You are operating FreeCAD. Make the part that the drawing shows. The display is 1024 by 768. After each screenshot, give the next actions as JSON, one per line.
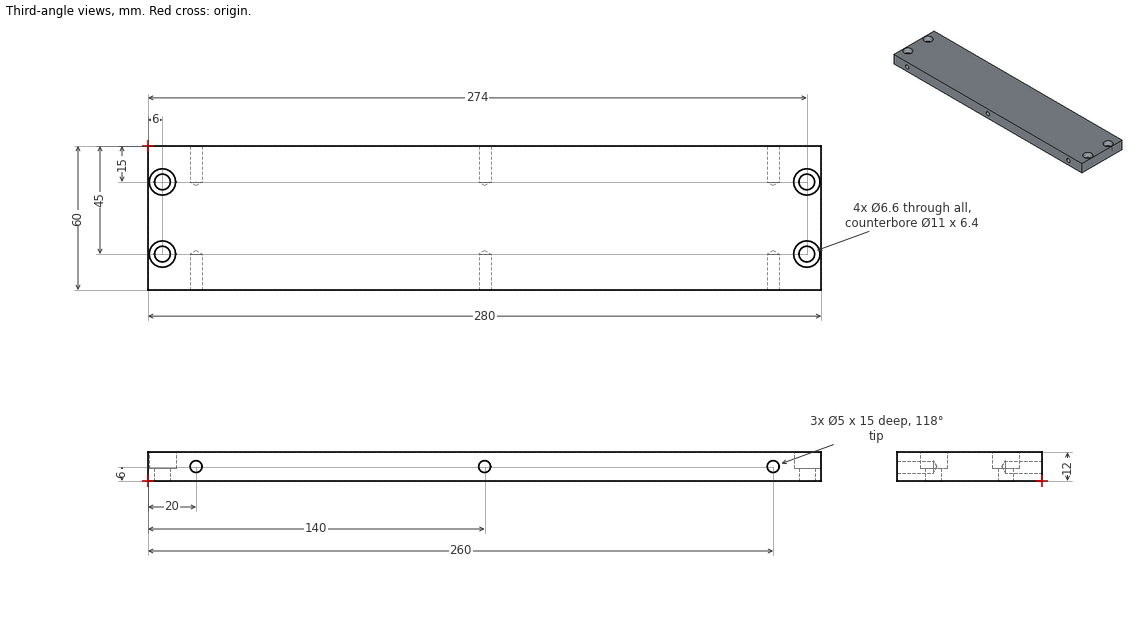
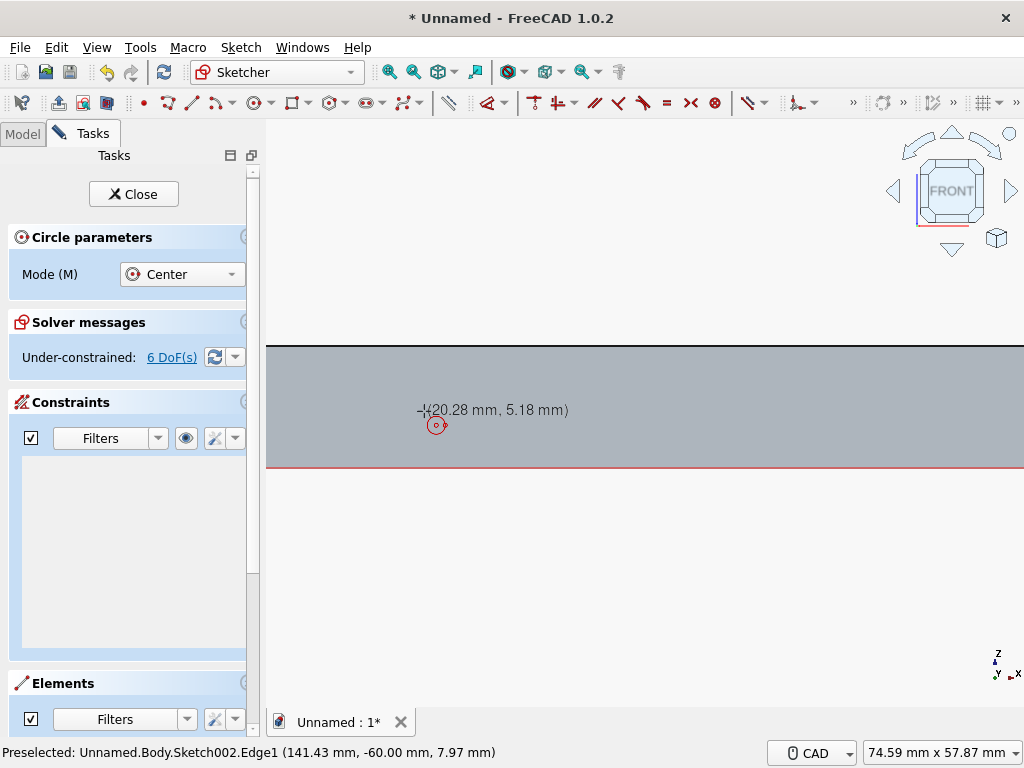
{"action": "scroll", "coordinate": [424, 411], "scroll_direction": "down", "scroll_amount": 10}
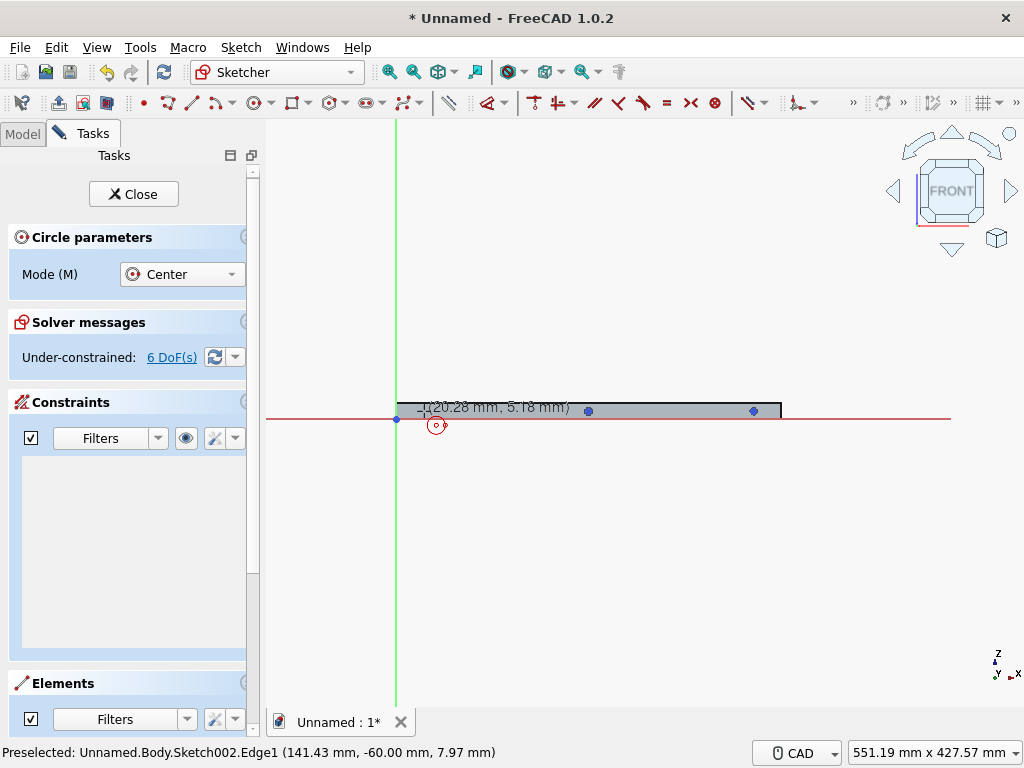
{"action": "scroll", "coordinate": [424, 411], "scroll_direction": "up", "scroll_amount": 4}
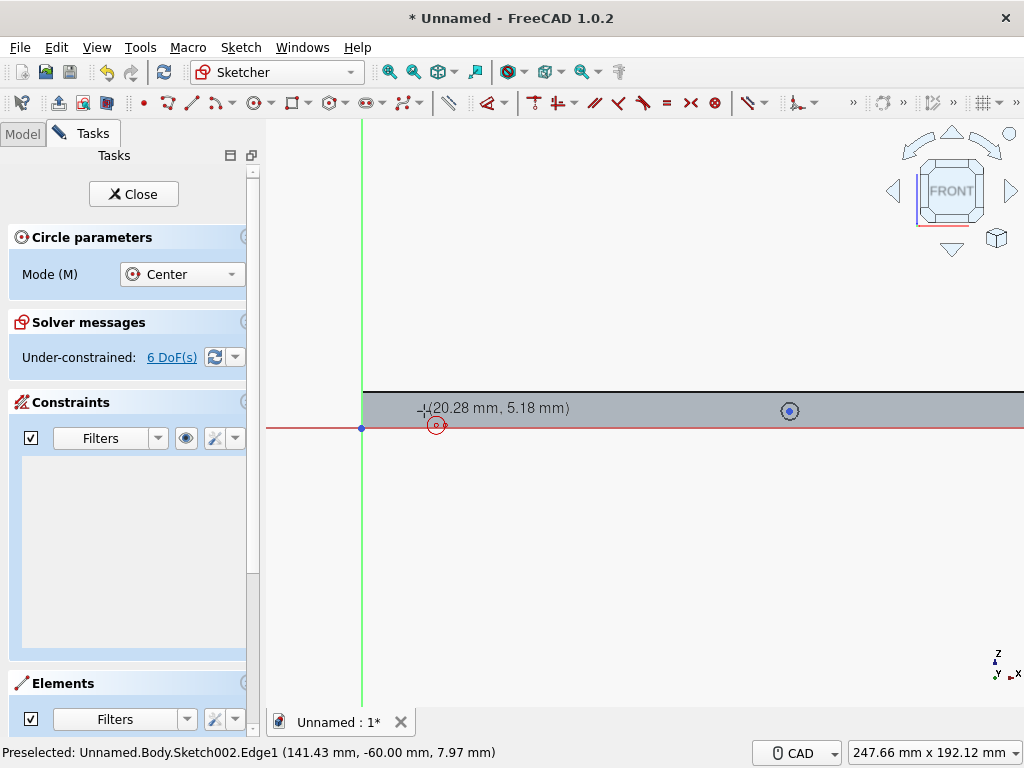
{"action": "left_click", "coordinate": [423, 410]}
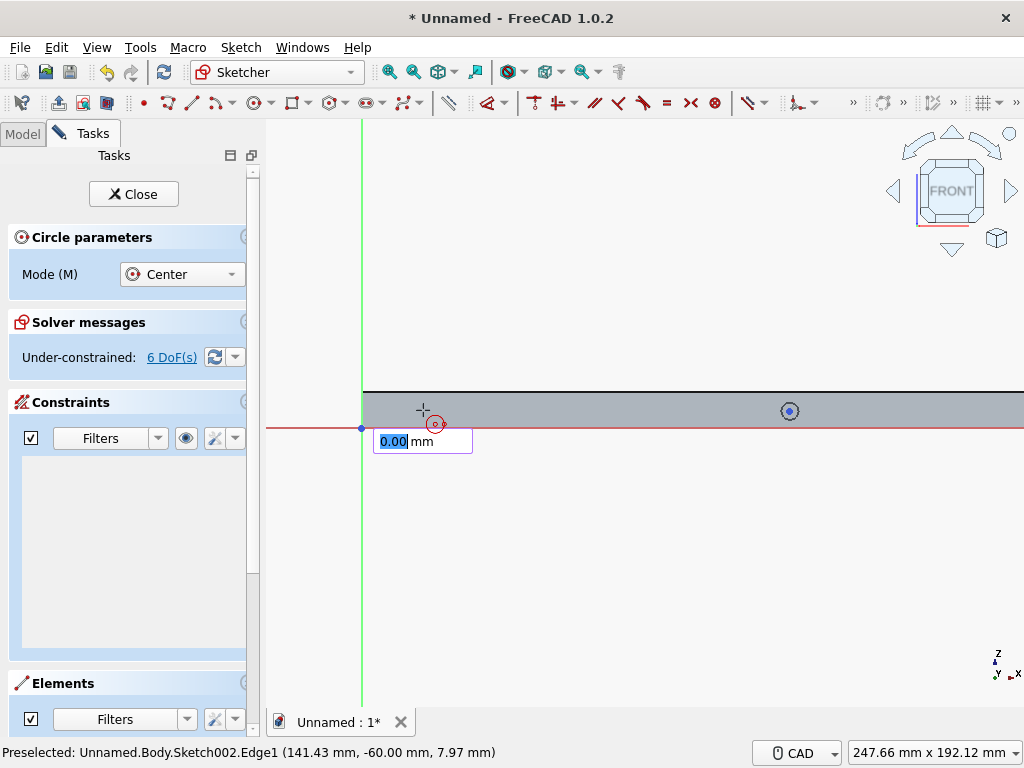
{"action": "scroll", "coordinate": [428, 405], "scroll_direction": "up", "scroll_amount": 4}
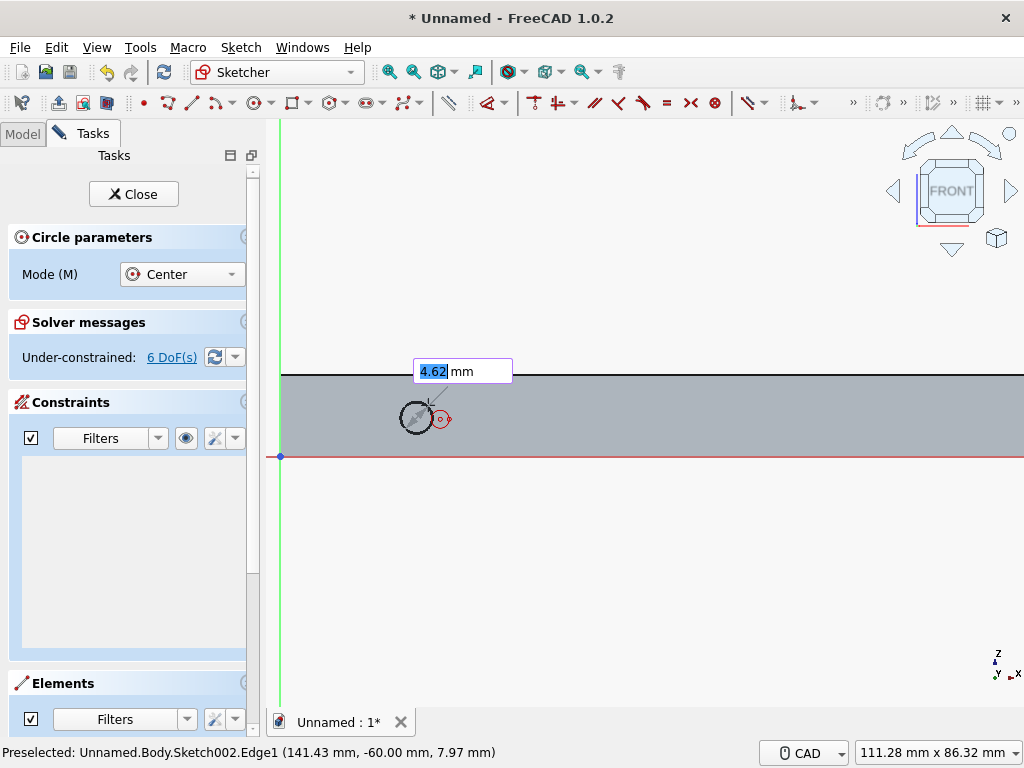
{"action": "left_click", "coordinate": [428, 404]}
{"action": "key", "text": "Escape"}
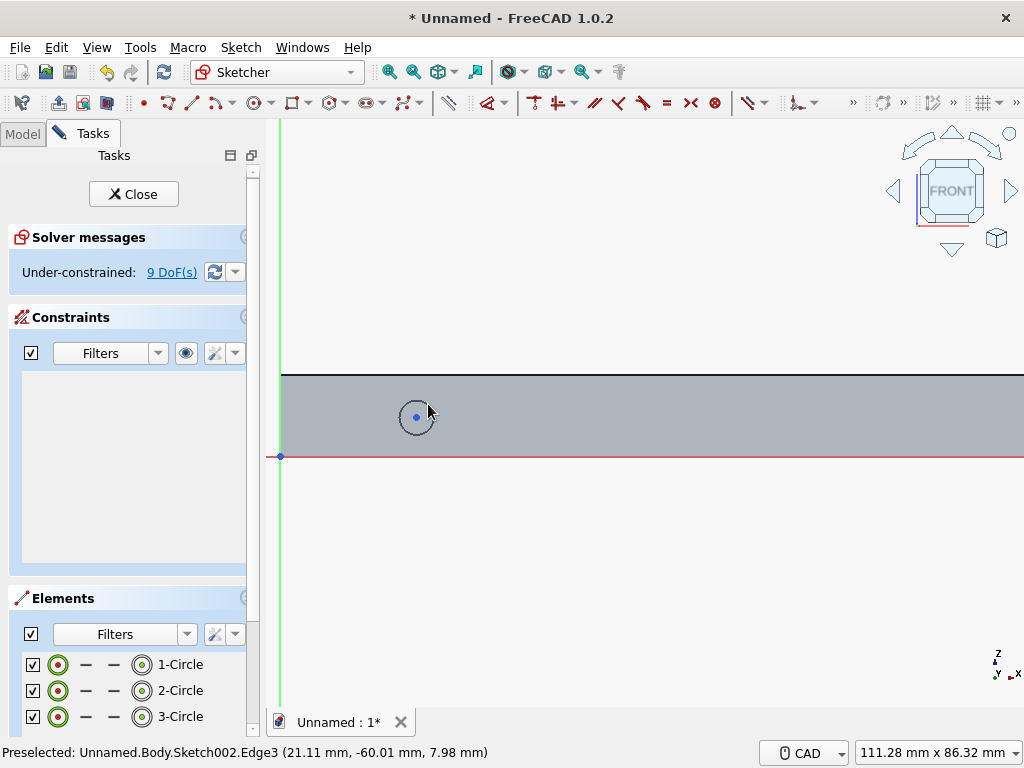
{"action": "scroll", "coordinate": [425, 409], "scroll_direction": "down", "scroll_amount": 8}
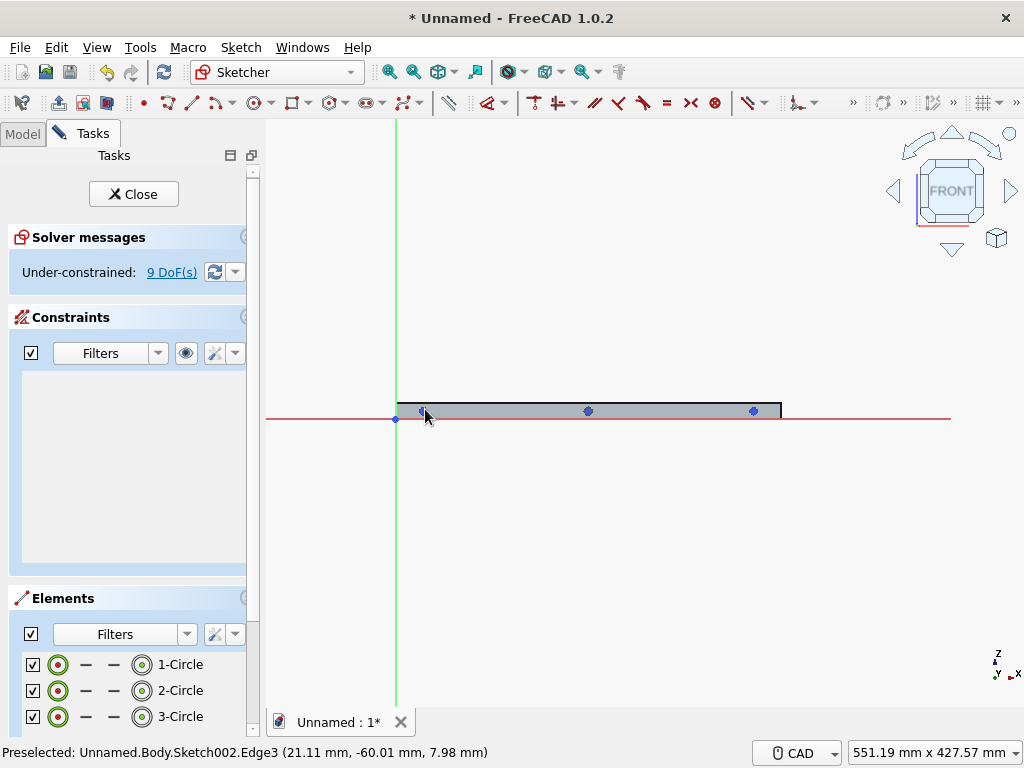
{"action": "scroll", "coordinate": [756, 409], "scroll_direction": "up", "scroll_amount": 8}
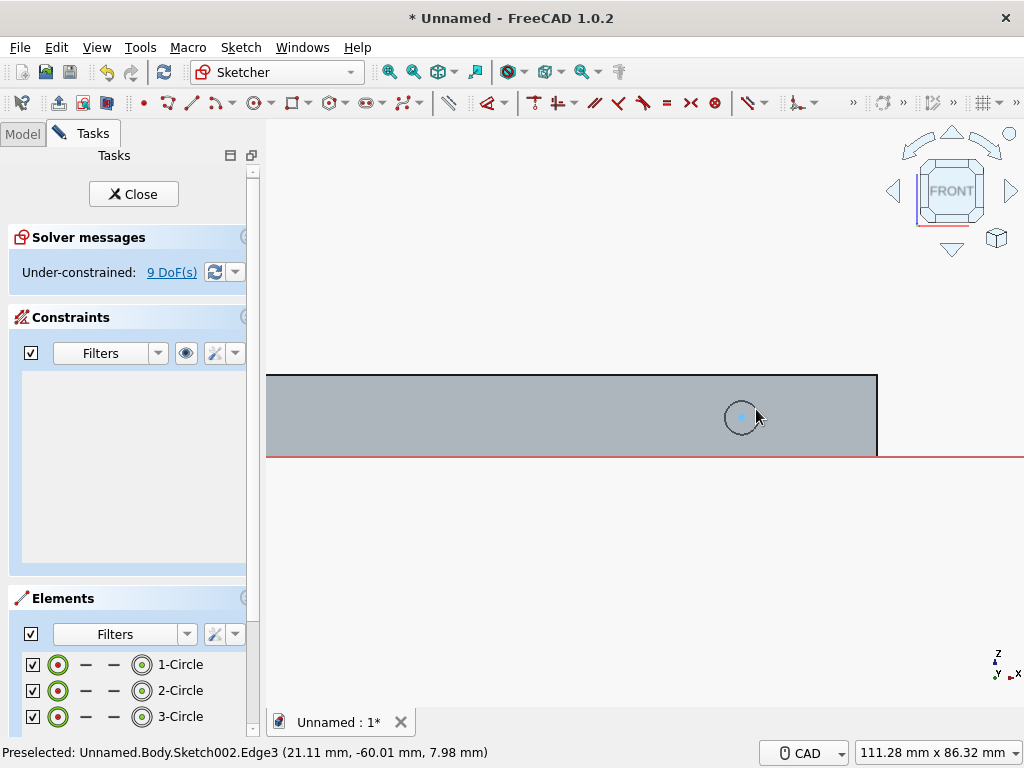
{"action": "left_click", "coordinate": [754, 406]}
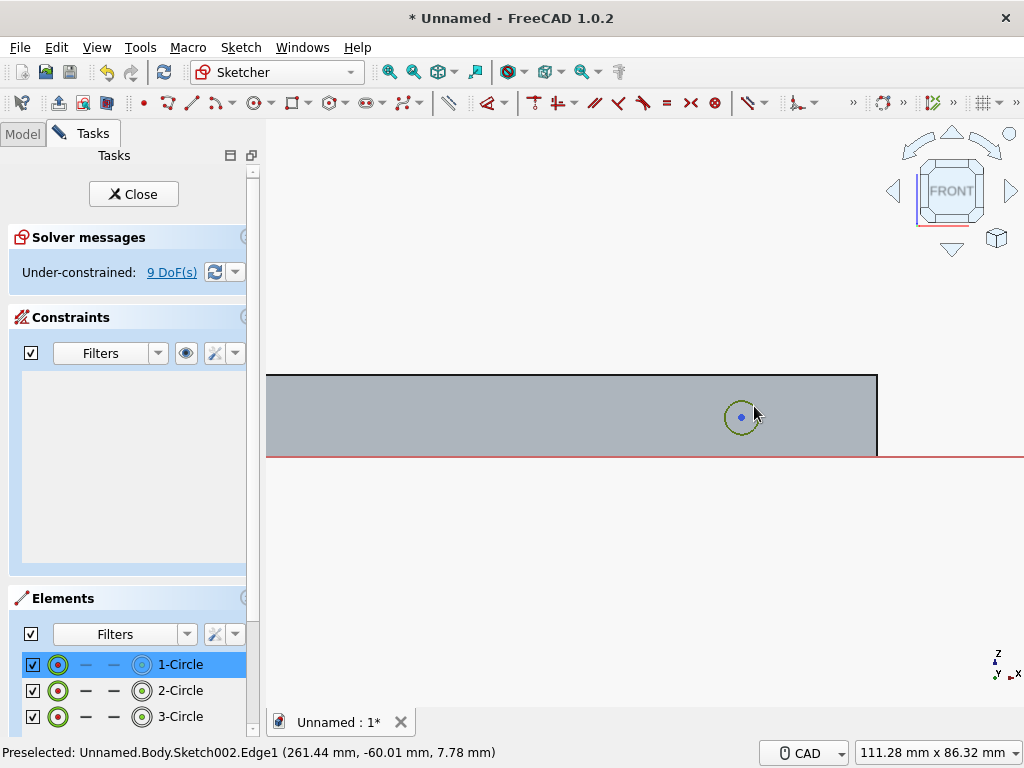
{"action": "scroll", "coordinate": [757, 409], "scroll_direction": "down", "scroll_amount": 8}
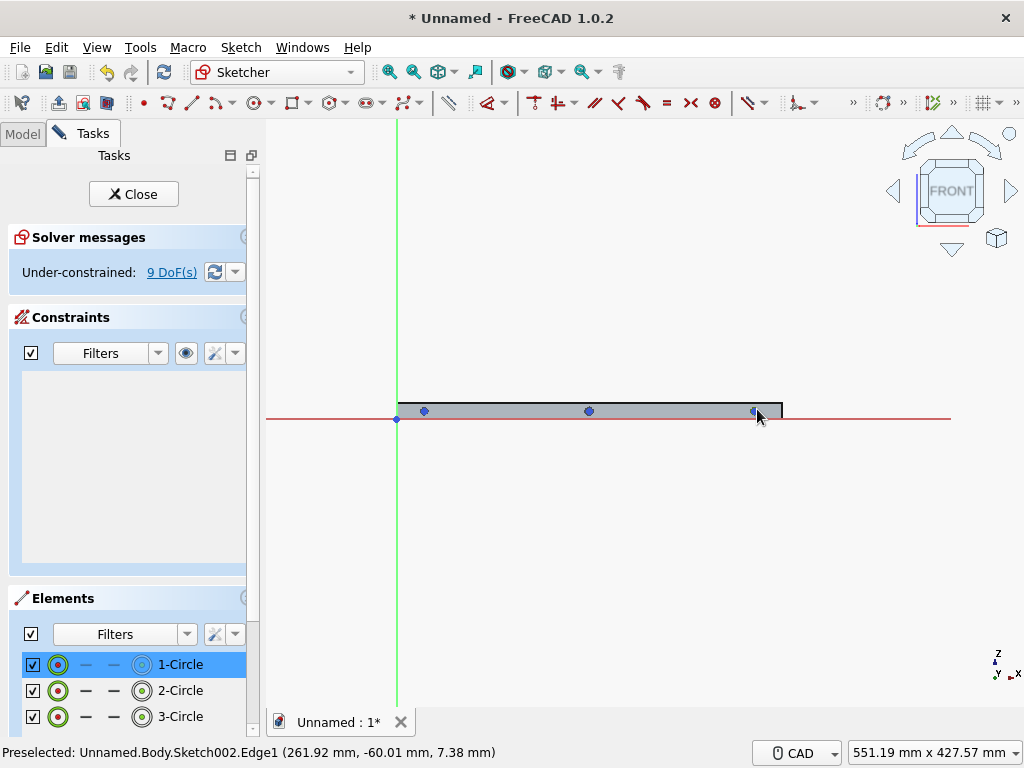
{"action": "scroll", "coordinate": [592, 409], "scroll_direction": "up", "scroll_amount": 7}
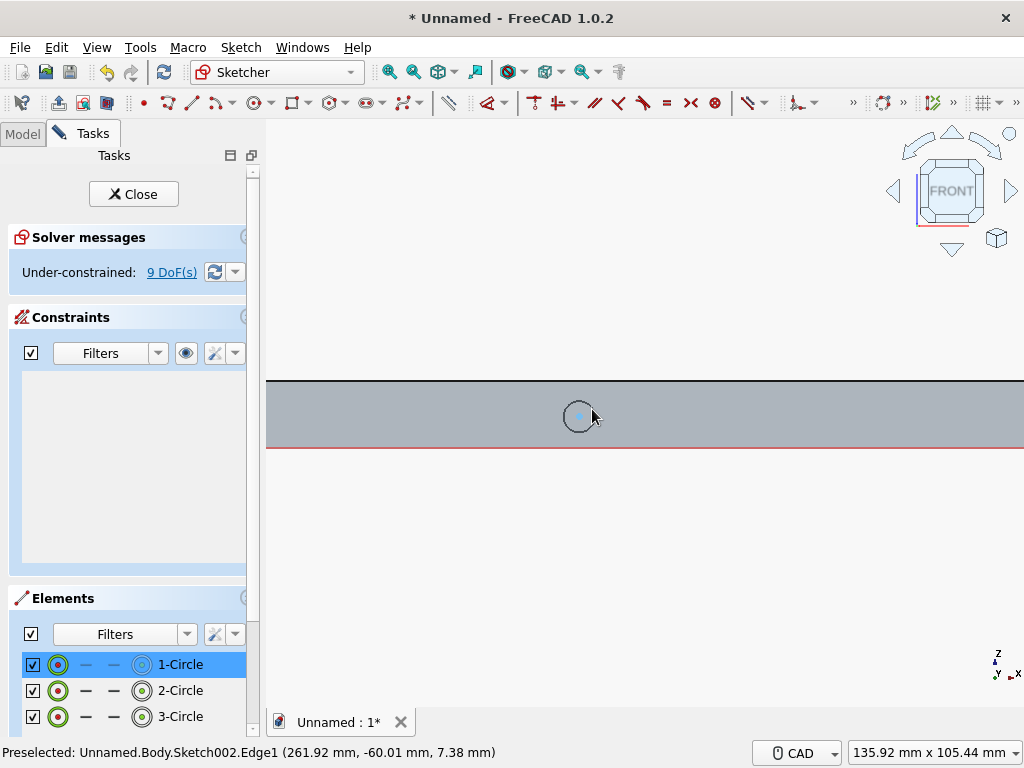
{"action": "left_click", "coordinate": [590, 406]}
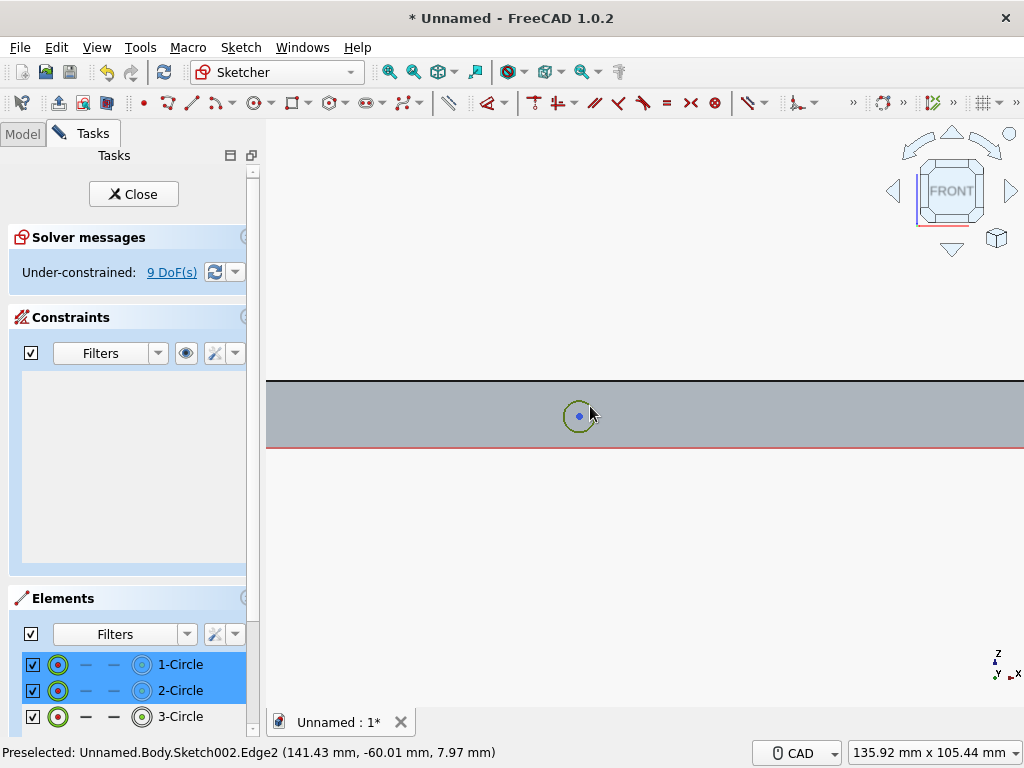
{"action": "scroll", "coordinate": [591, 409], "scroll_direction": "down", "scroll_amount": 7}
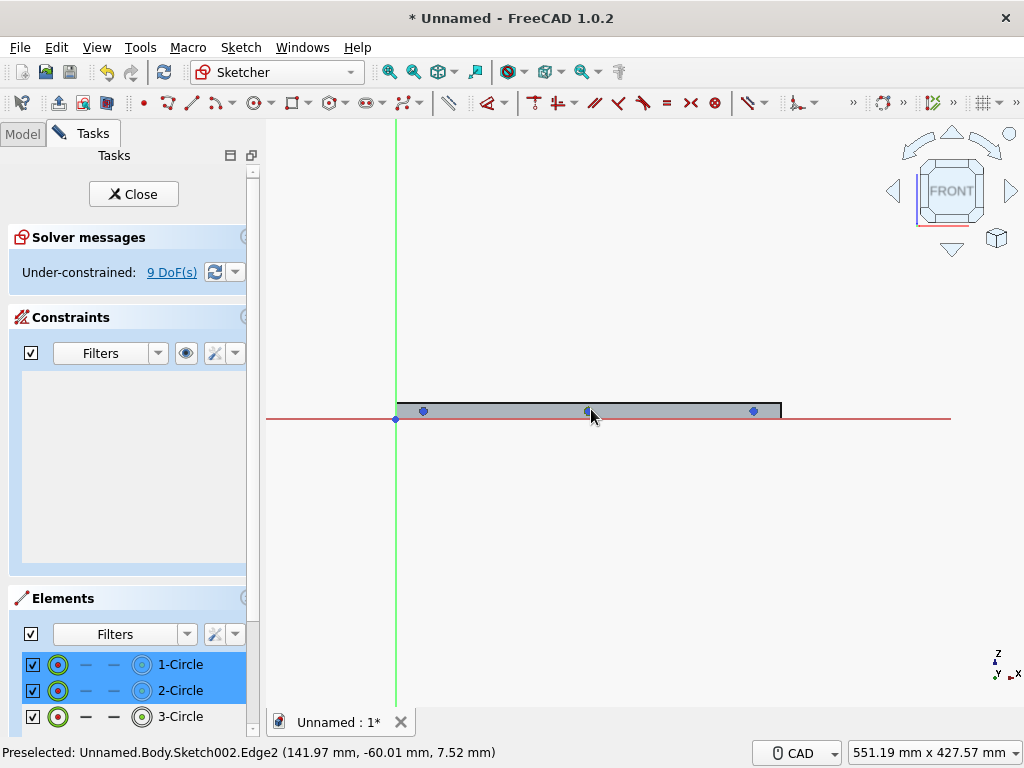
{"action": "scroll", "coordinate": [426, 409], "scroll_direction": "up", "scroll_amount": 7}